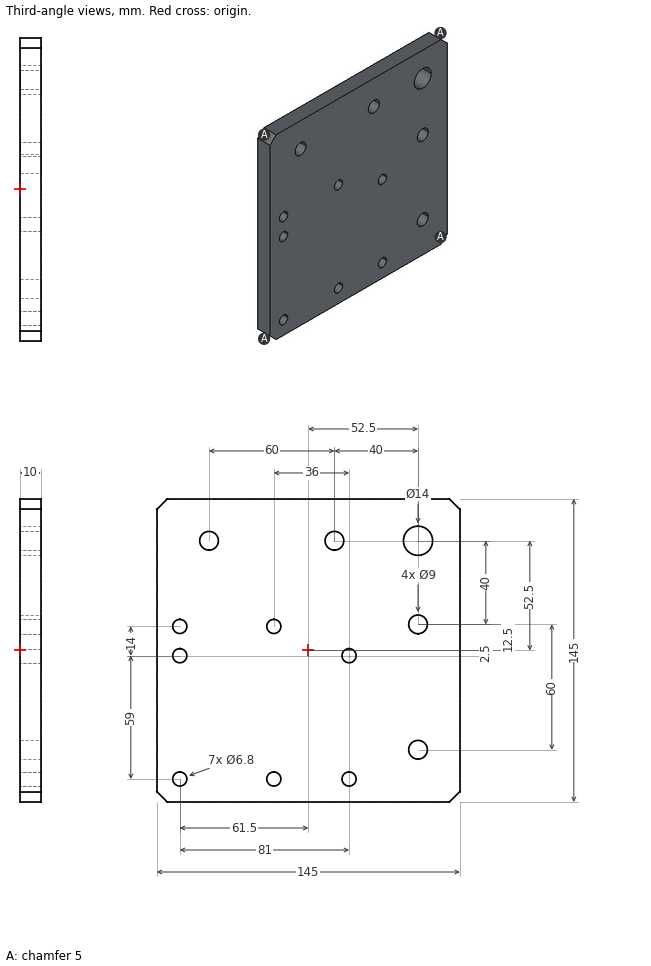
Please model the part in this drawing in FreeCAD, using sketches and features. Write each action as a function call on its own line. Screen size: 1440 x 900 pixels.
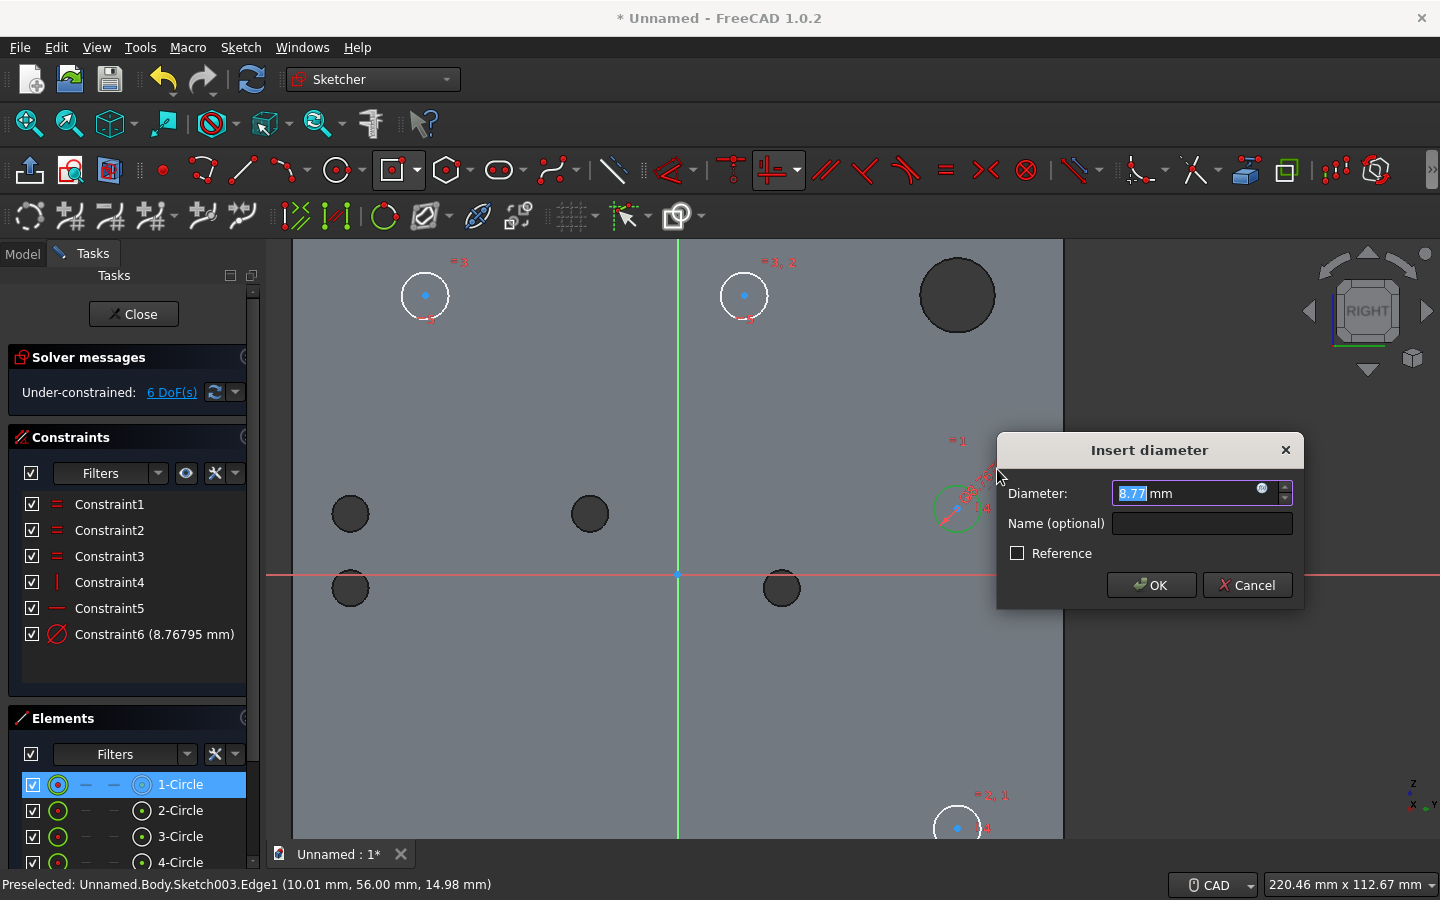
text(9)
key(Return)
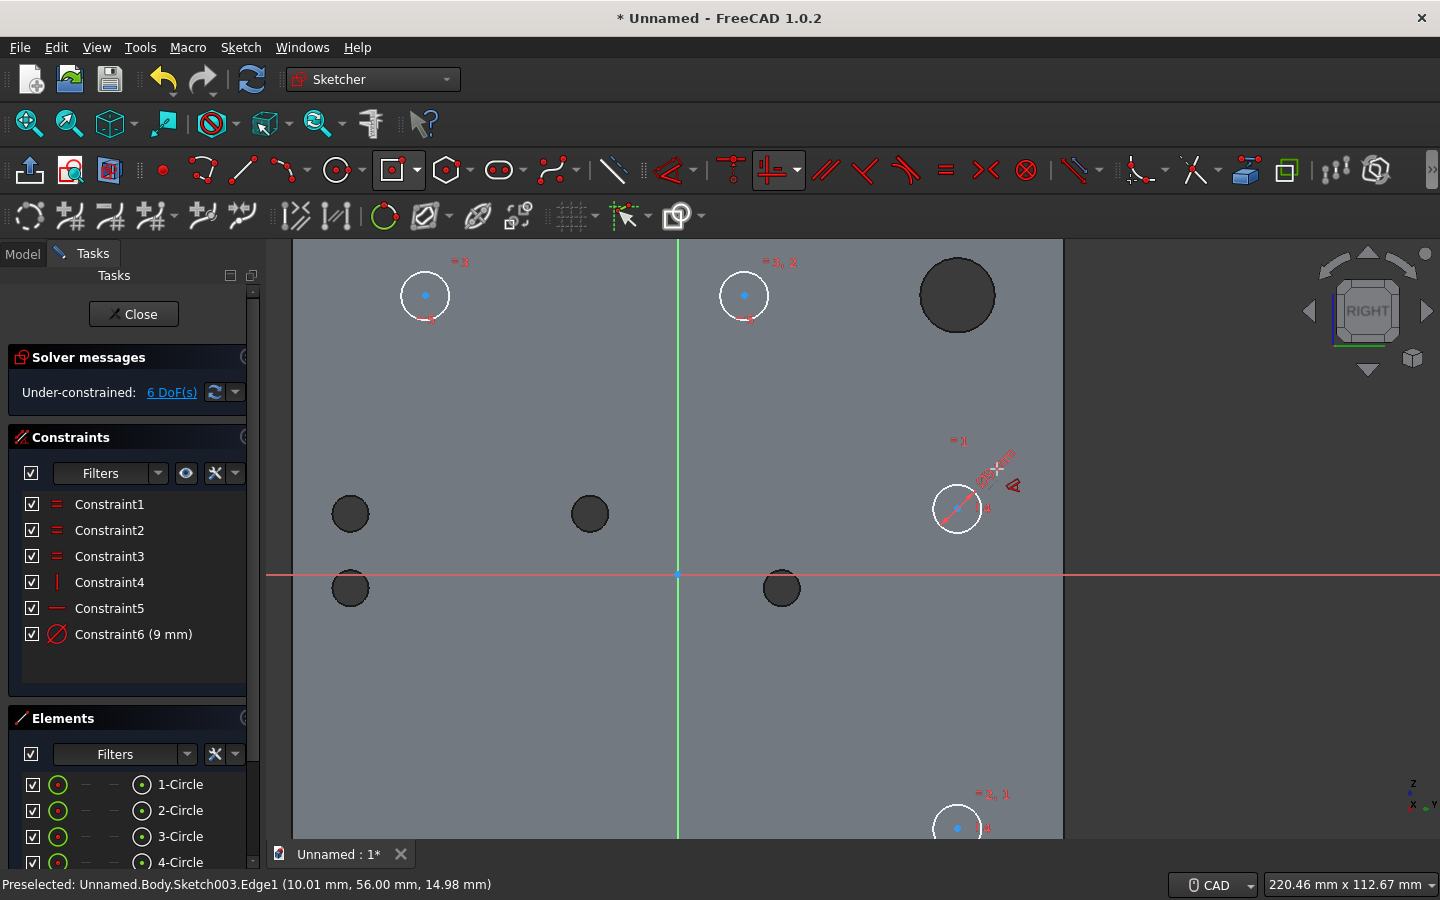
click(957, 509)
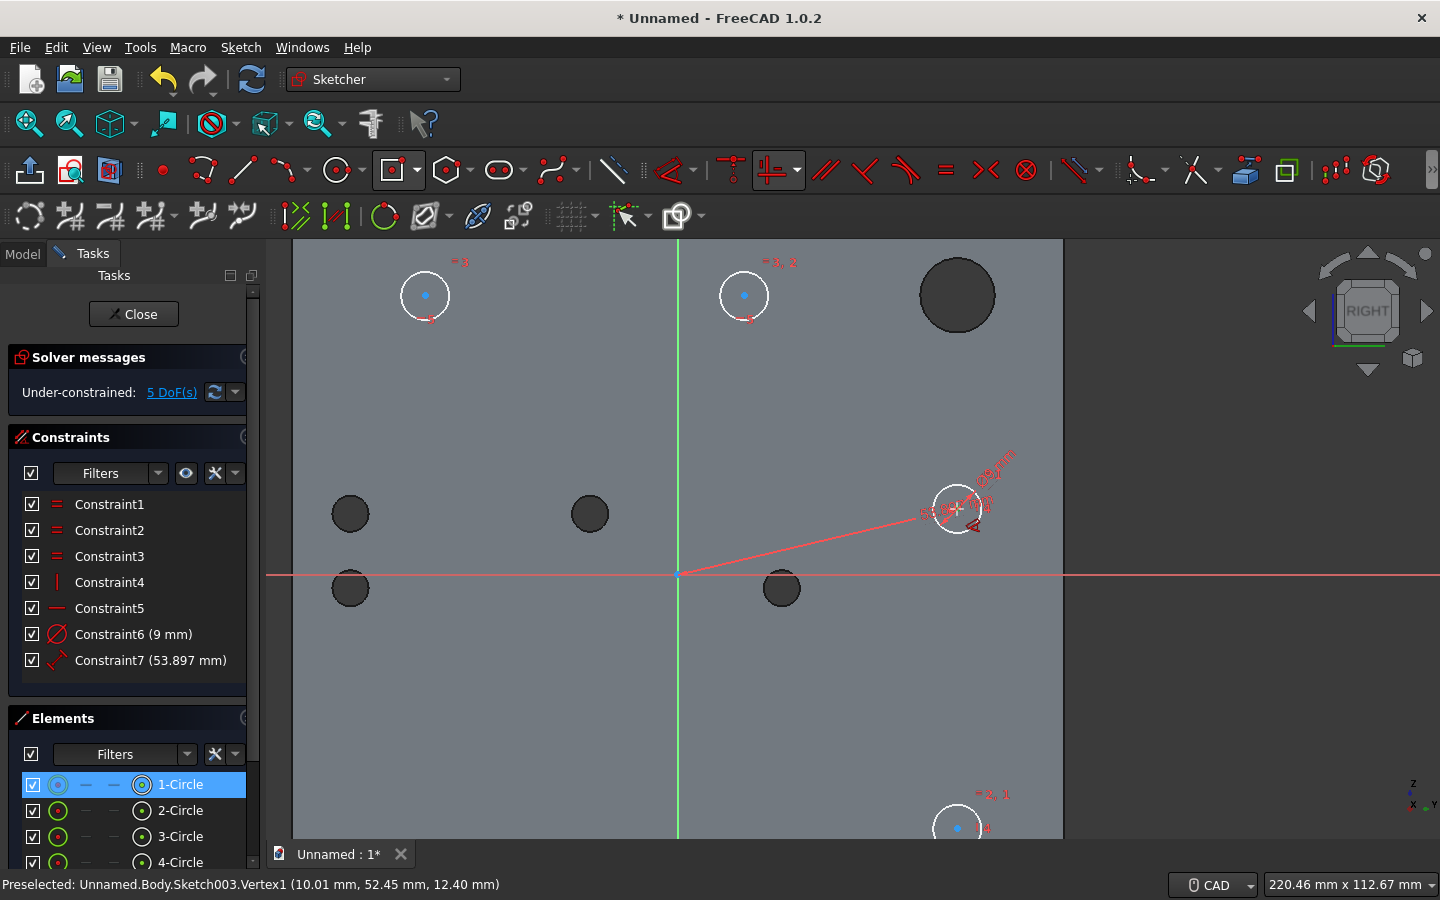
scroll(974, 493, down, 2)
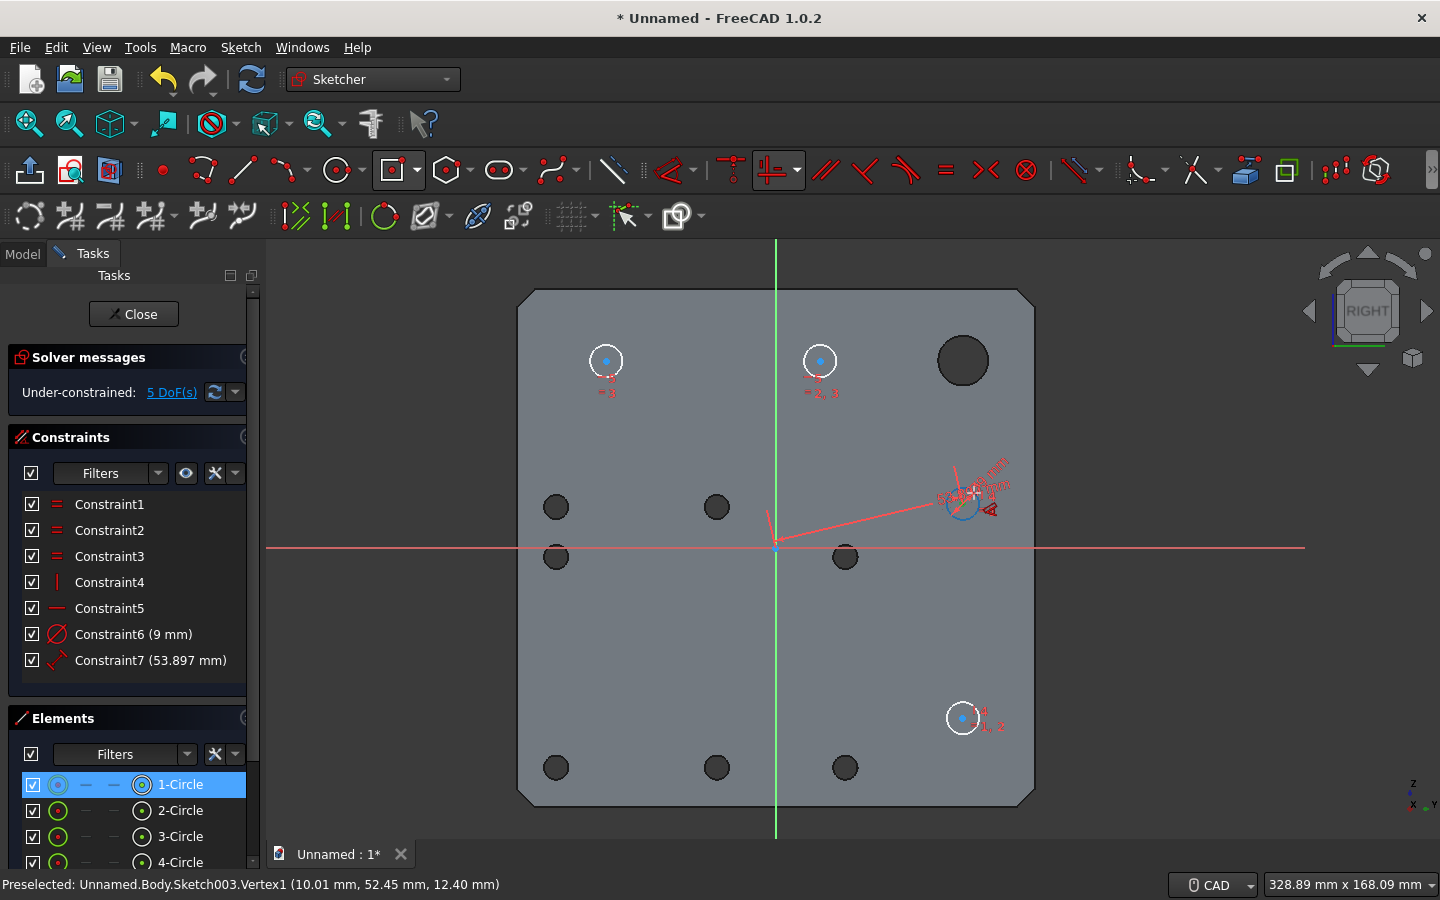
click(963, 718)
click(997, 611)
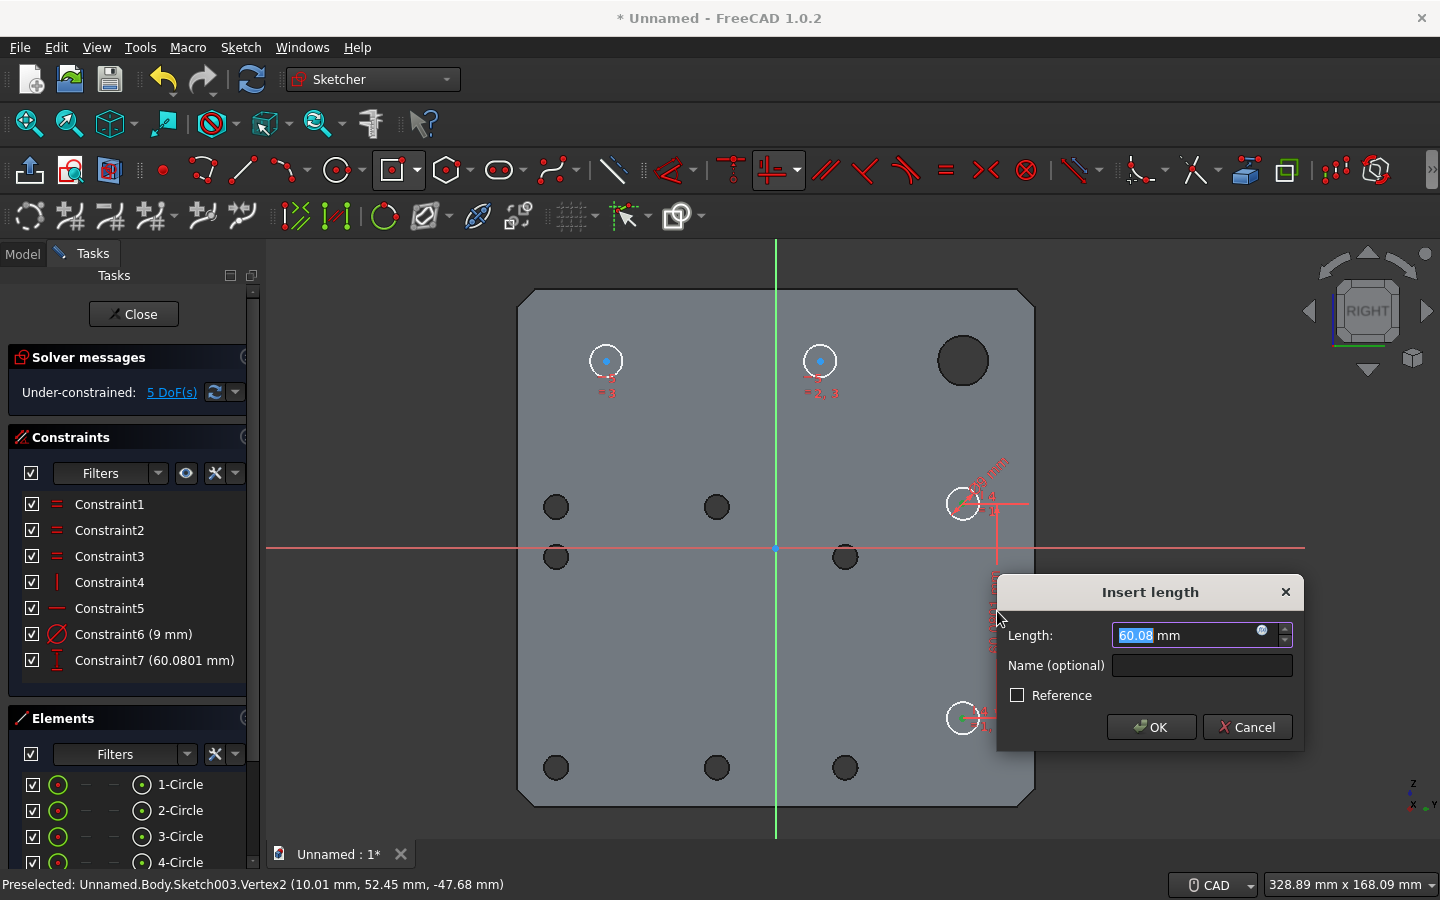
text(60)
key(Return)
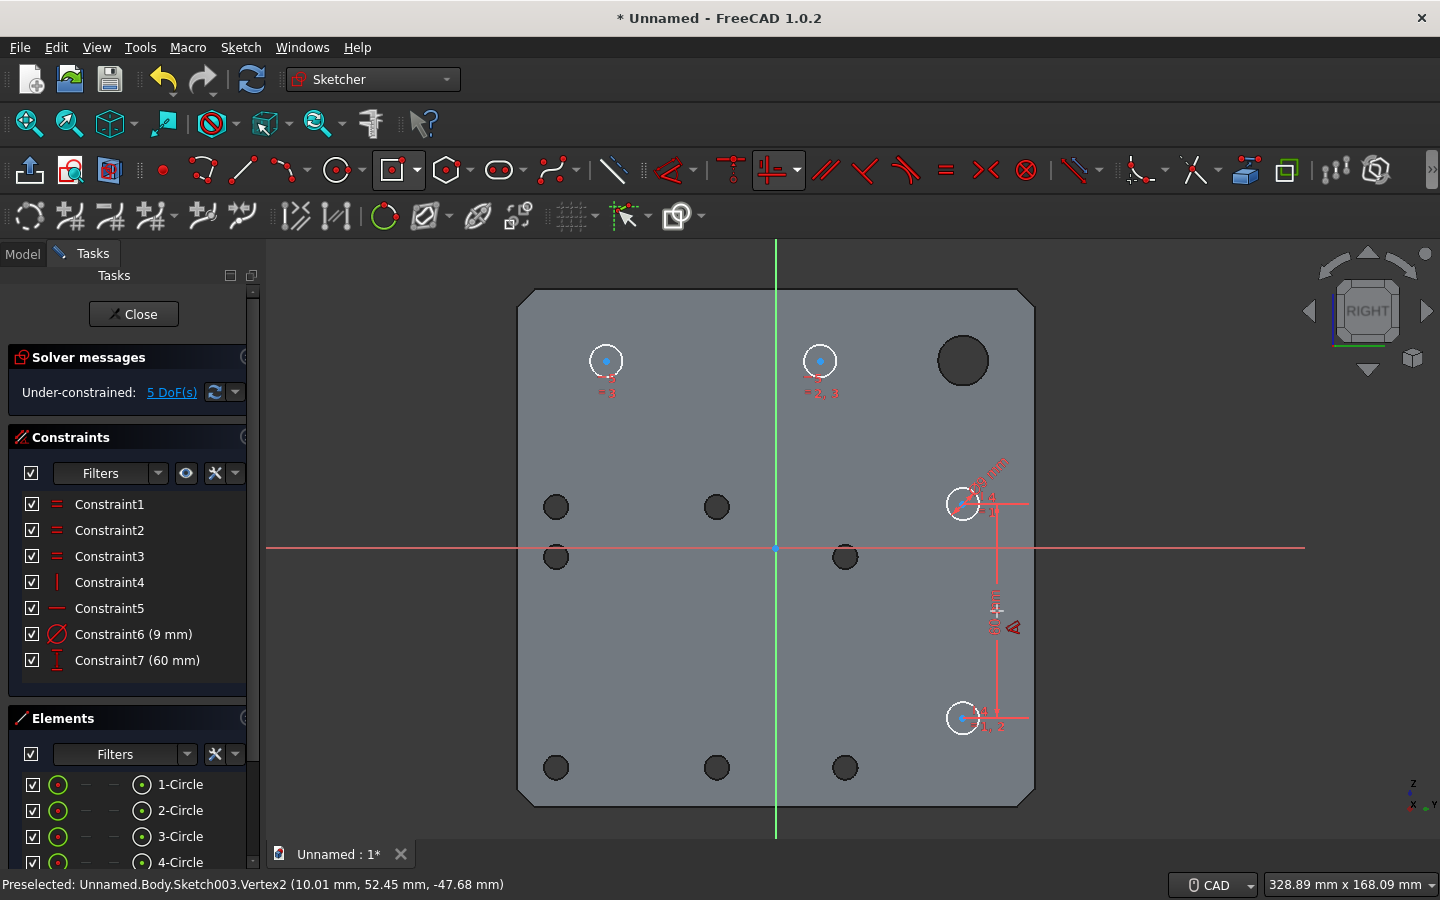
click(963, 504)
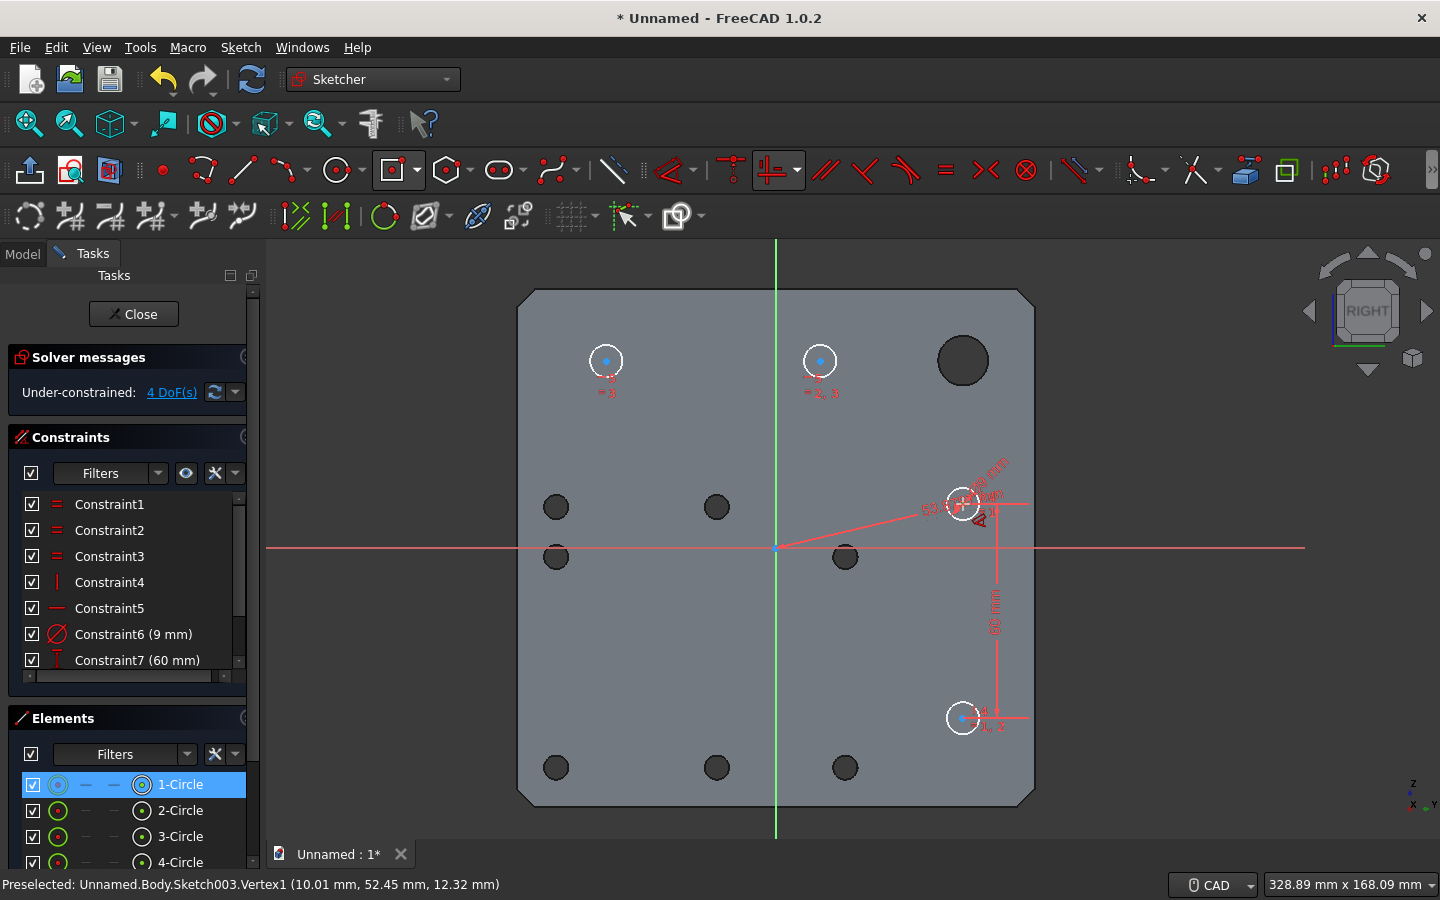
click(820, 361)
click(892, 327)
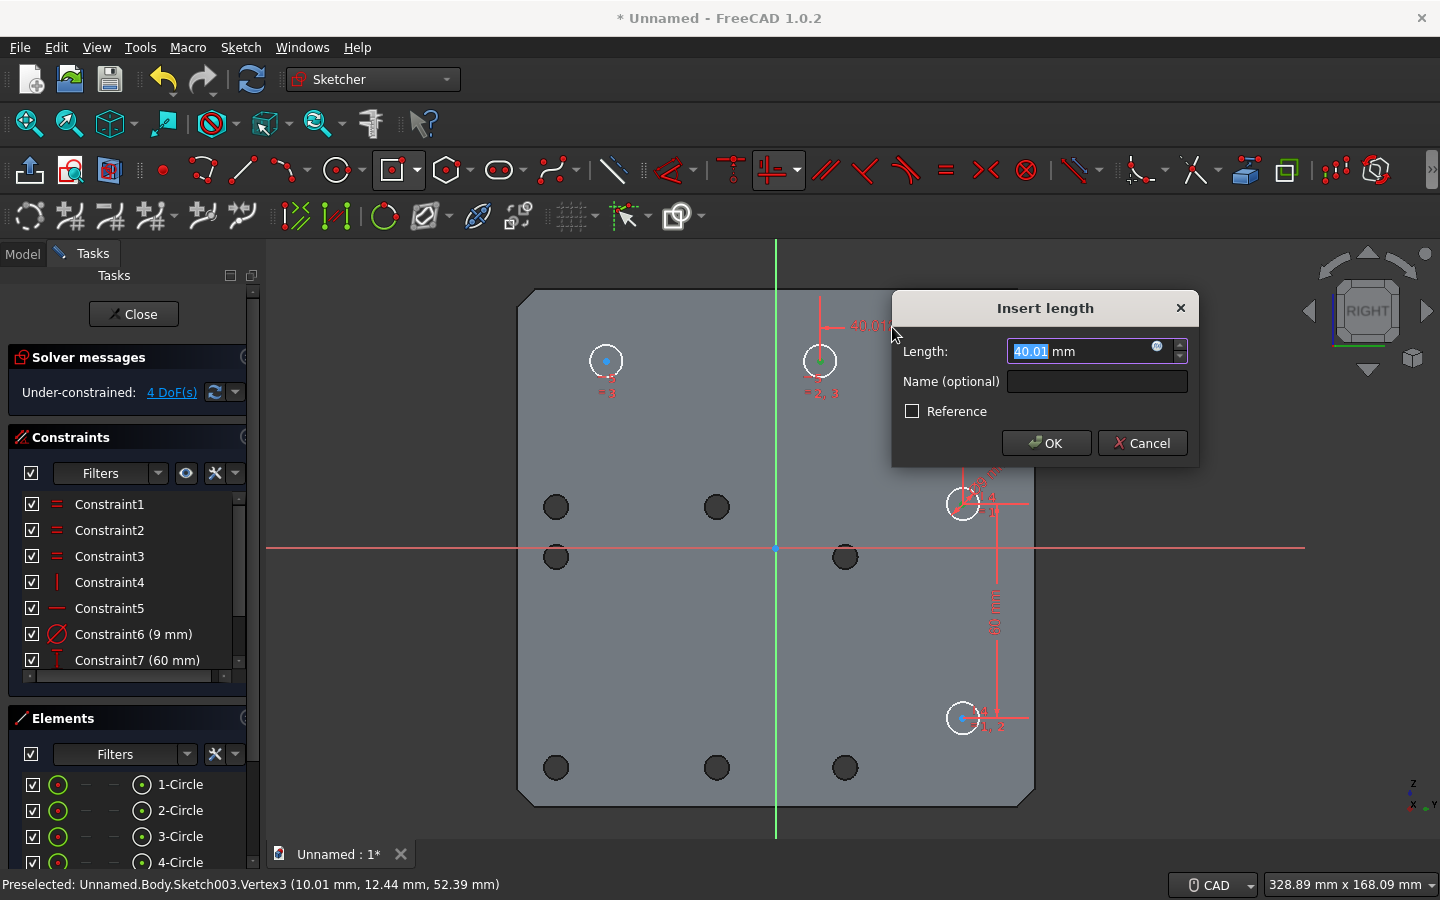
text(40)
key(Return)